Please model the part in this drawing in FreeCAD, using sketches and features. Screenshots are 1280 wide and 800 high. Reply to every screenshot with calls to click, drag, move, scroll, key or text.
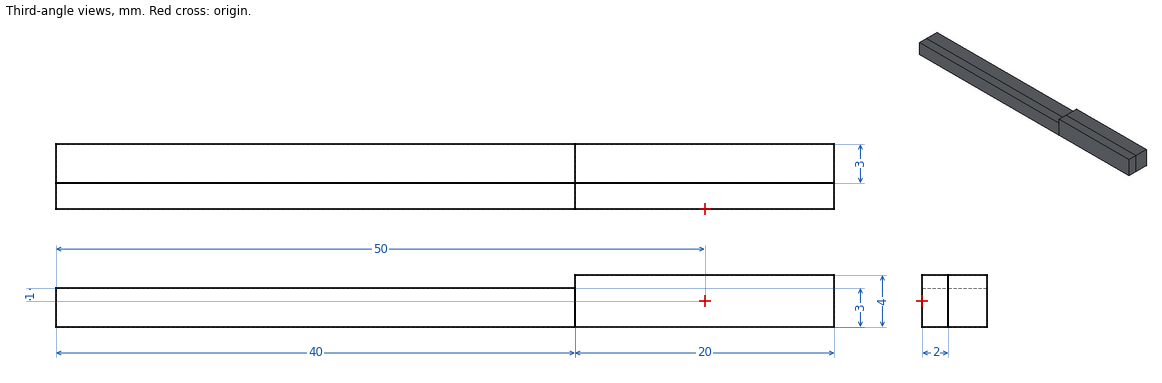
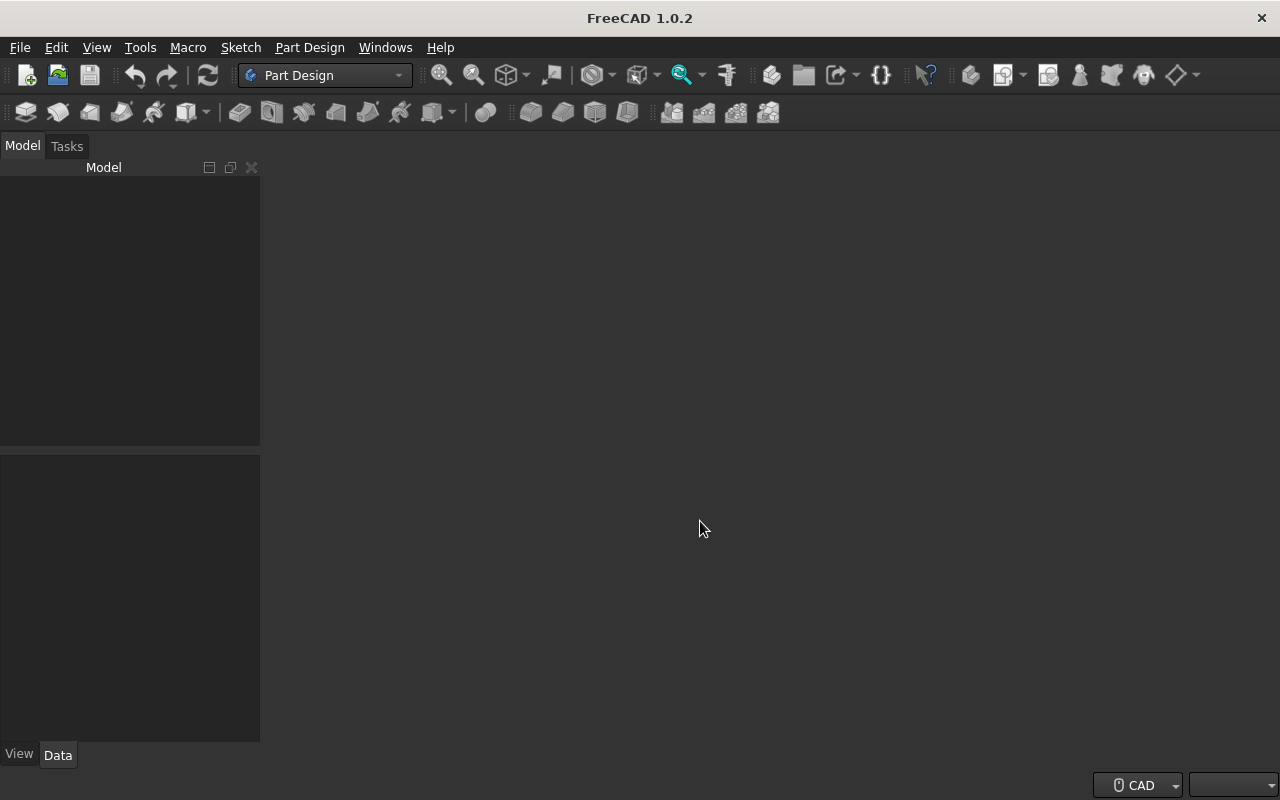
click(26, 76)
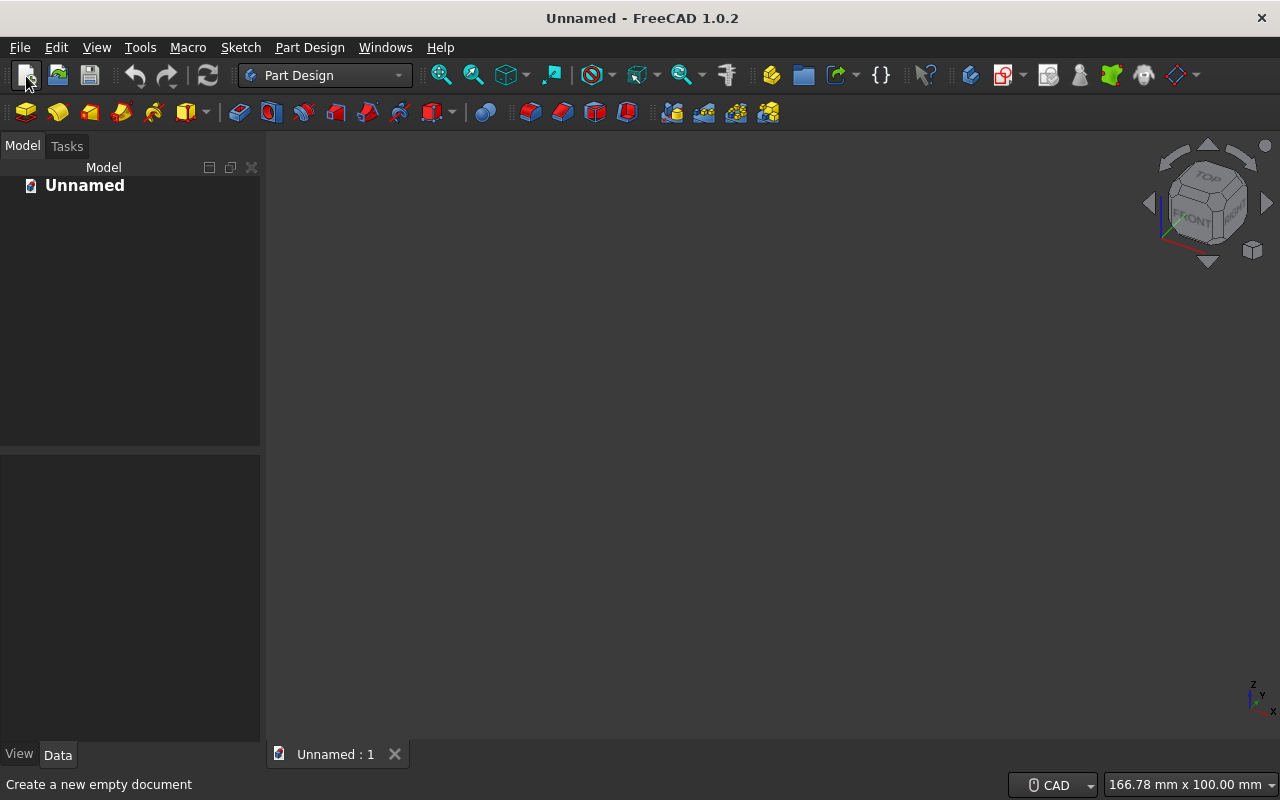
click(1004, 76)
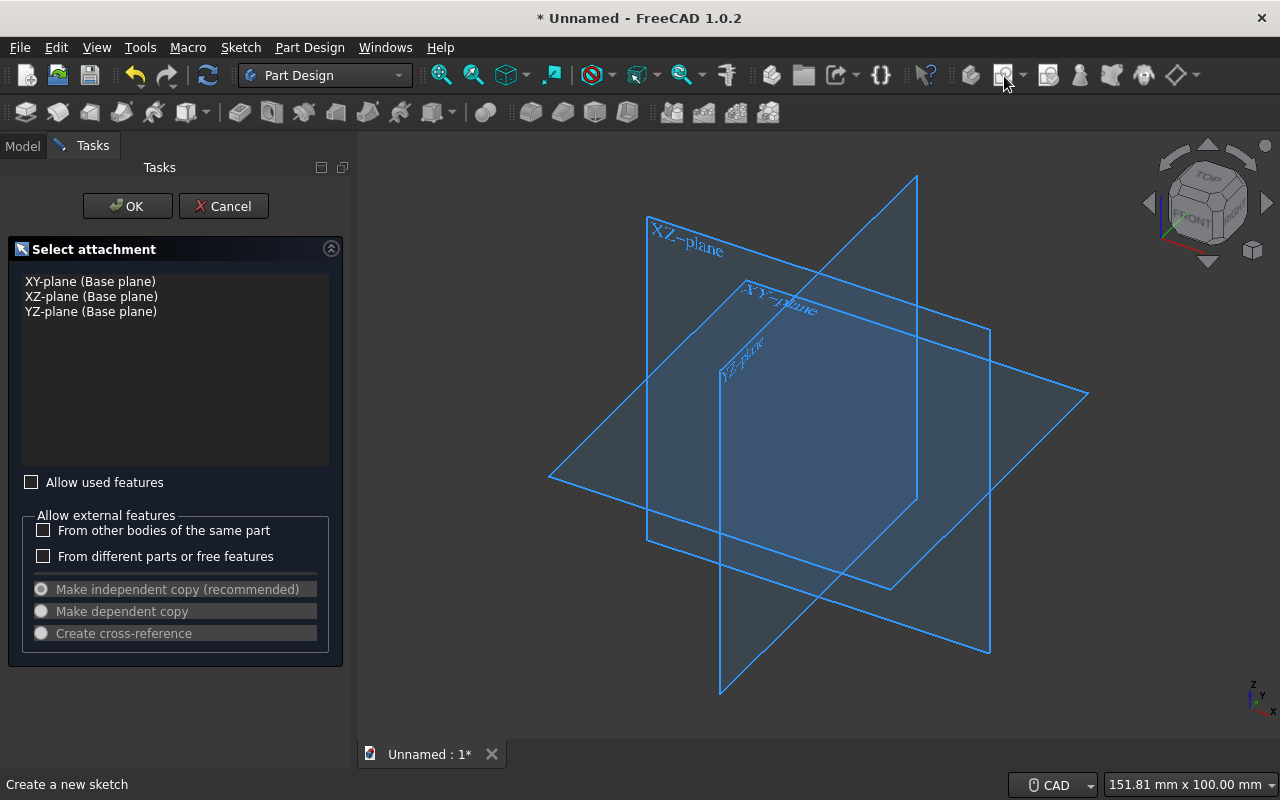
click(82, 296)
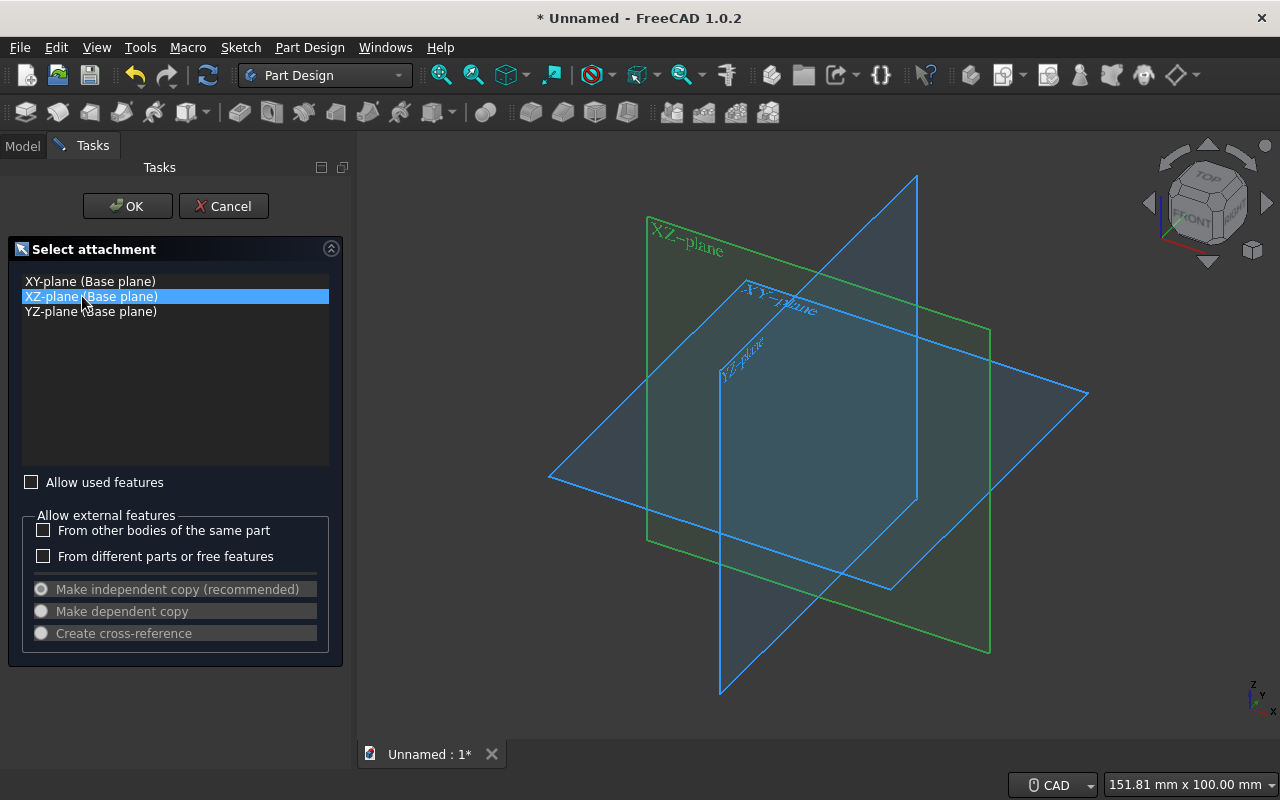
click(128, 206)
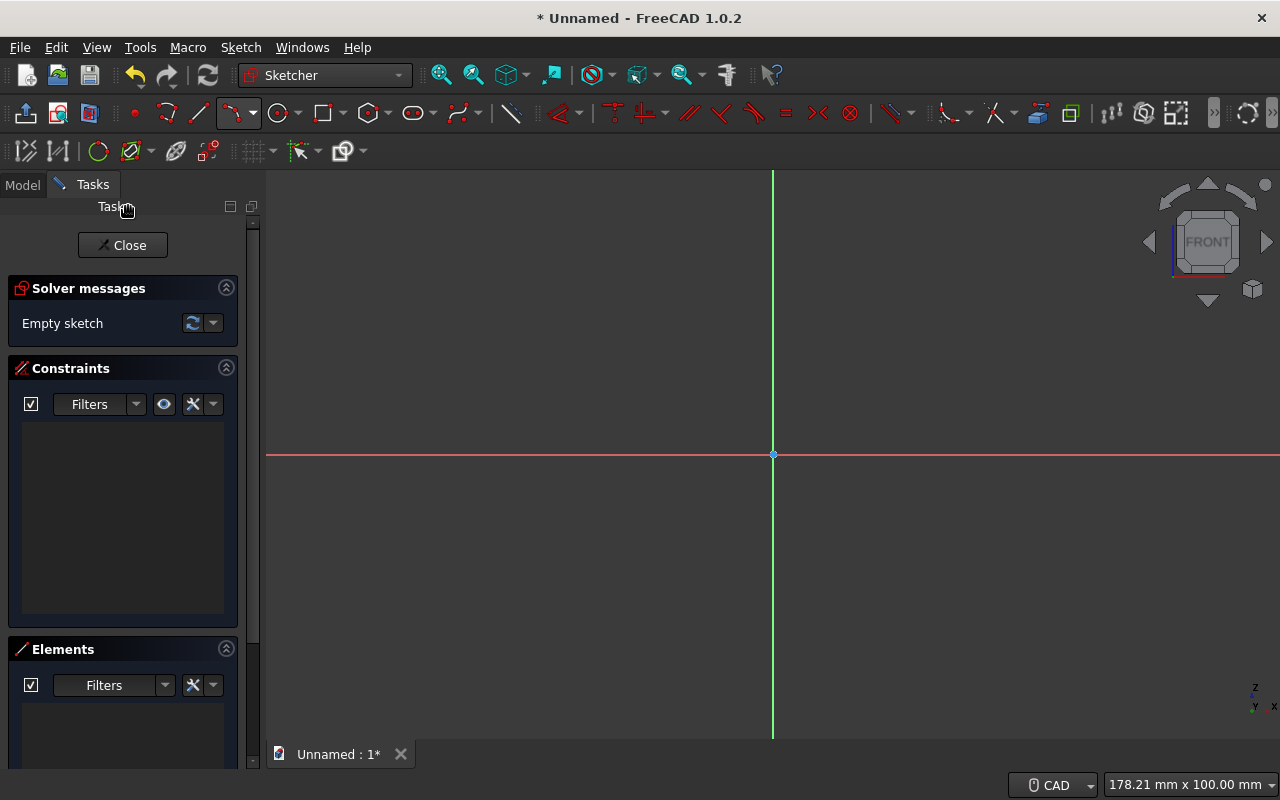
scroll(790, 454, up, 8)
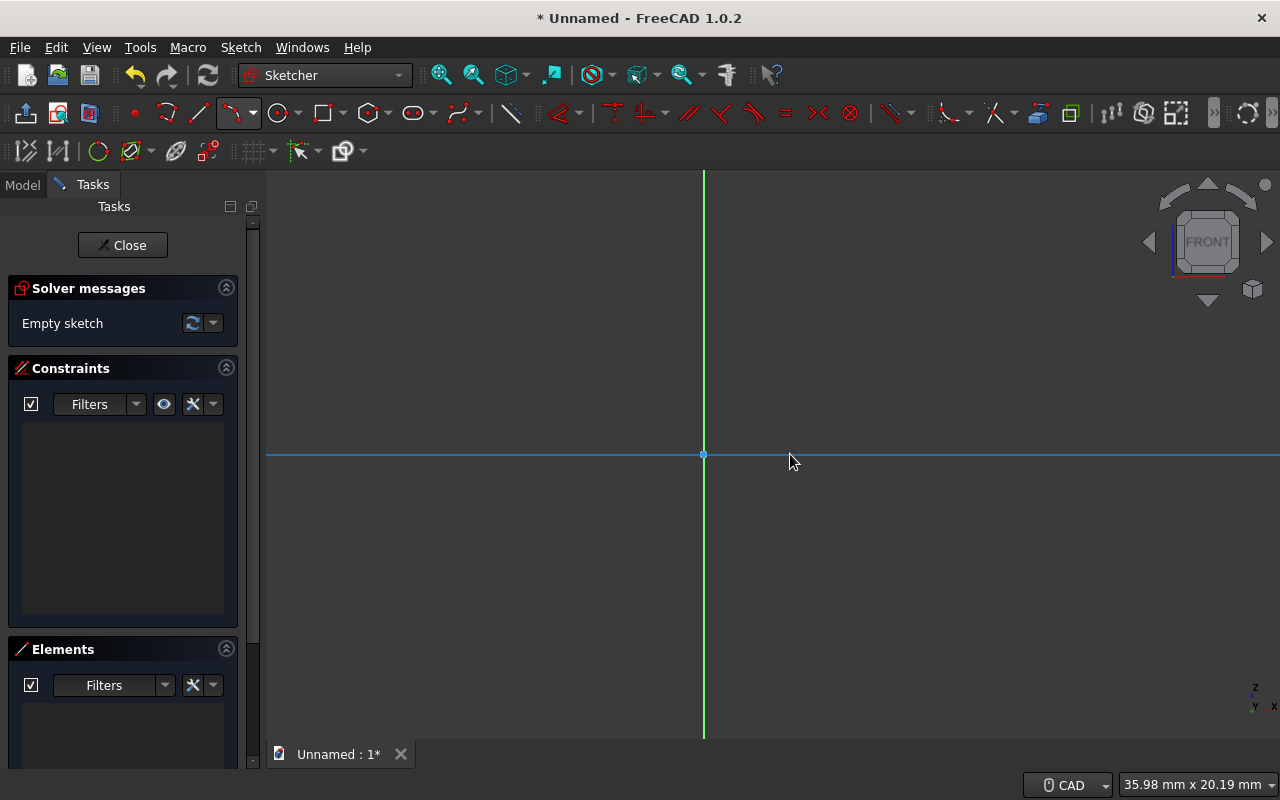
click(346, 114)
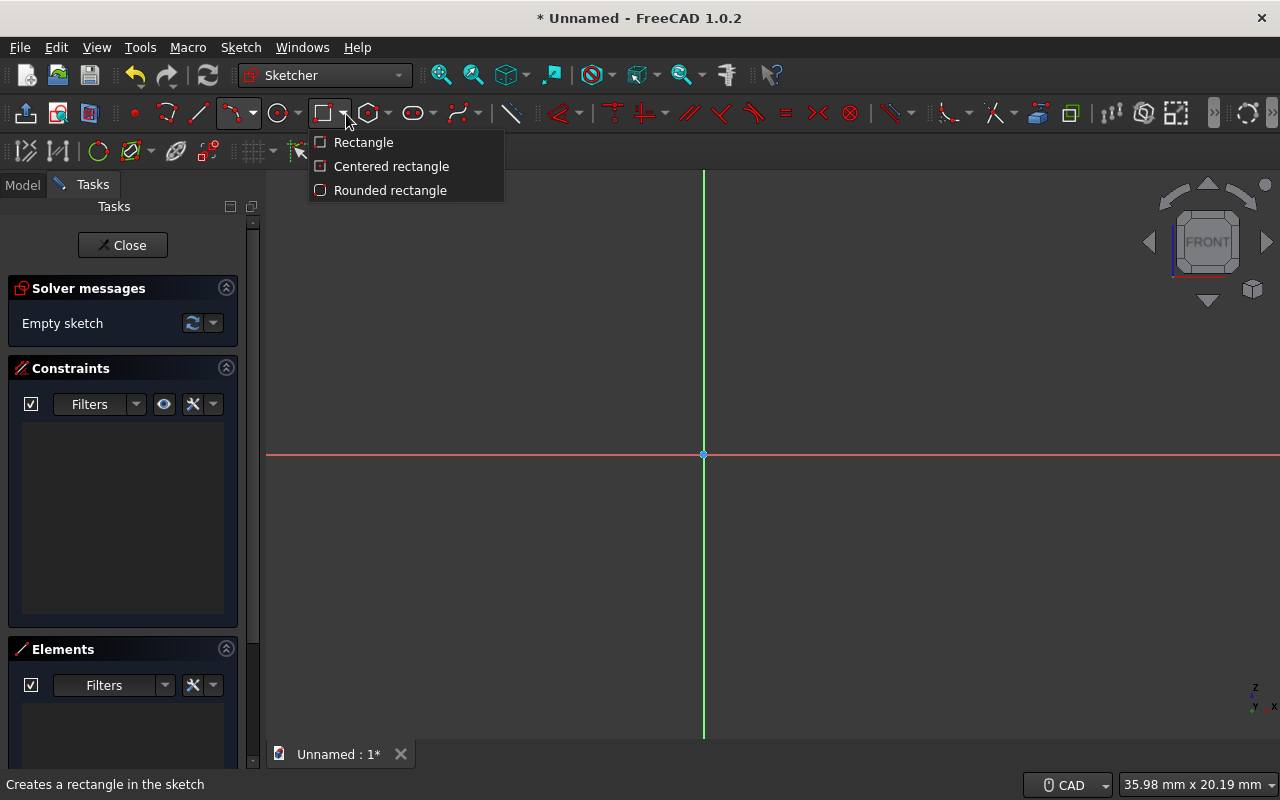
click(406, 166)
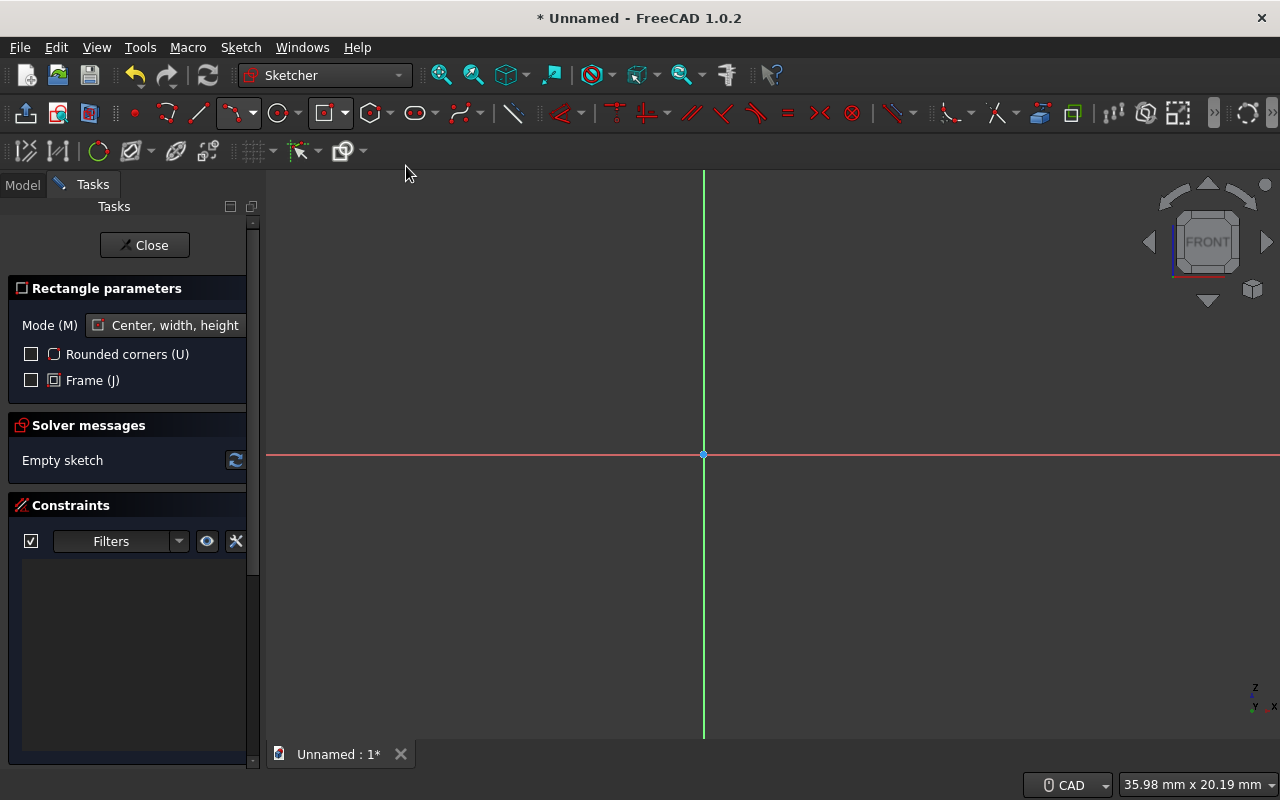
click(704, 454)
move(986, 398)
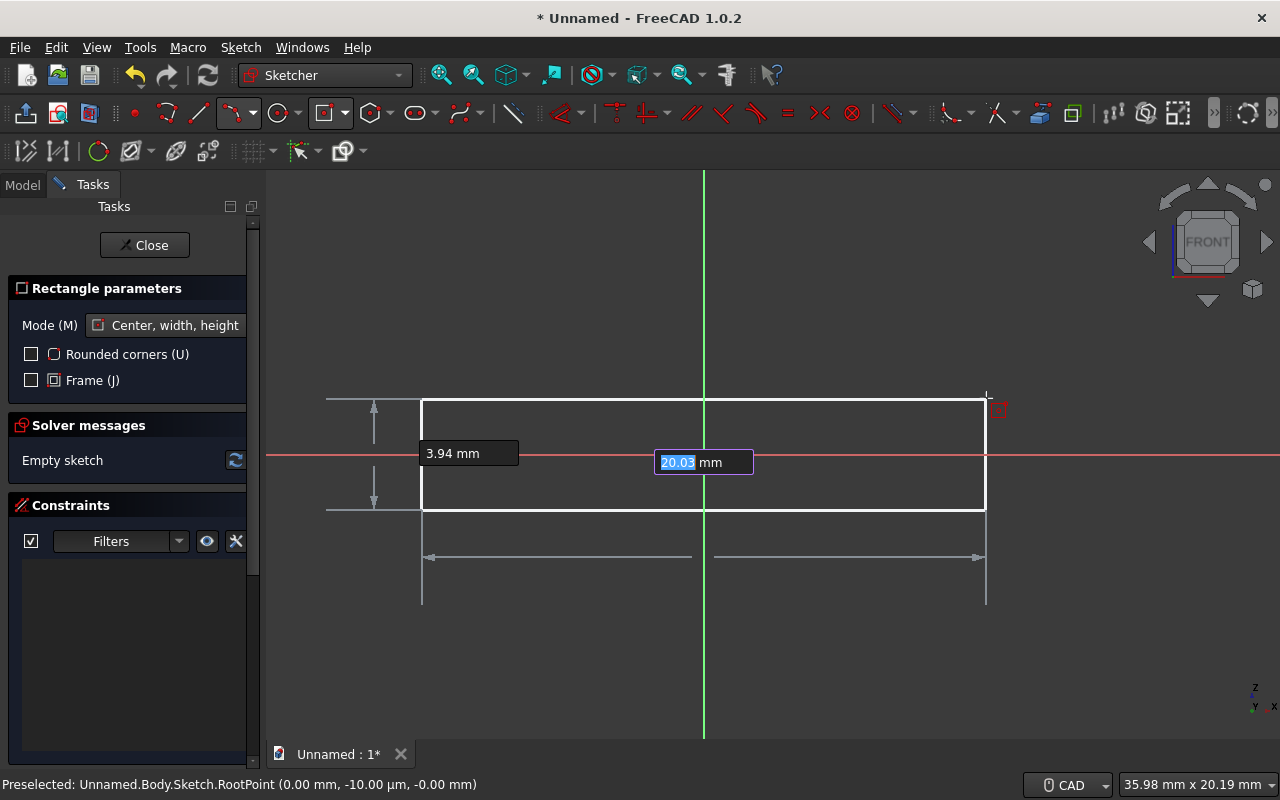
text(20)
key(Tab)
text(4)
key(Return)
key(Escape)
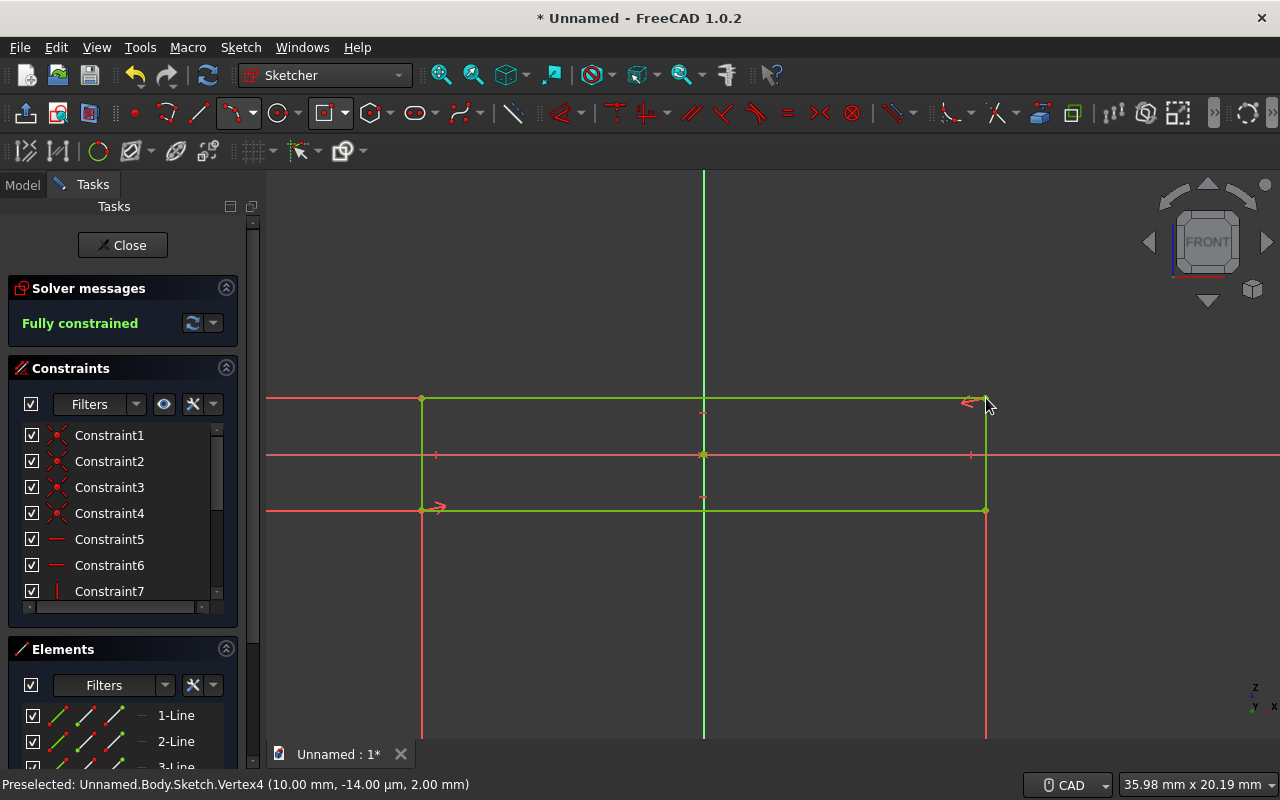
click(123, 245)